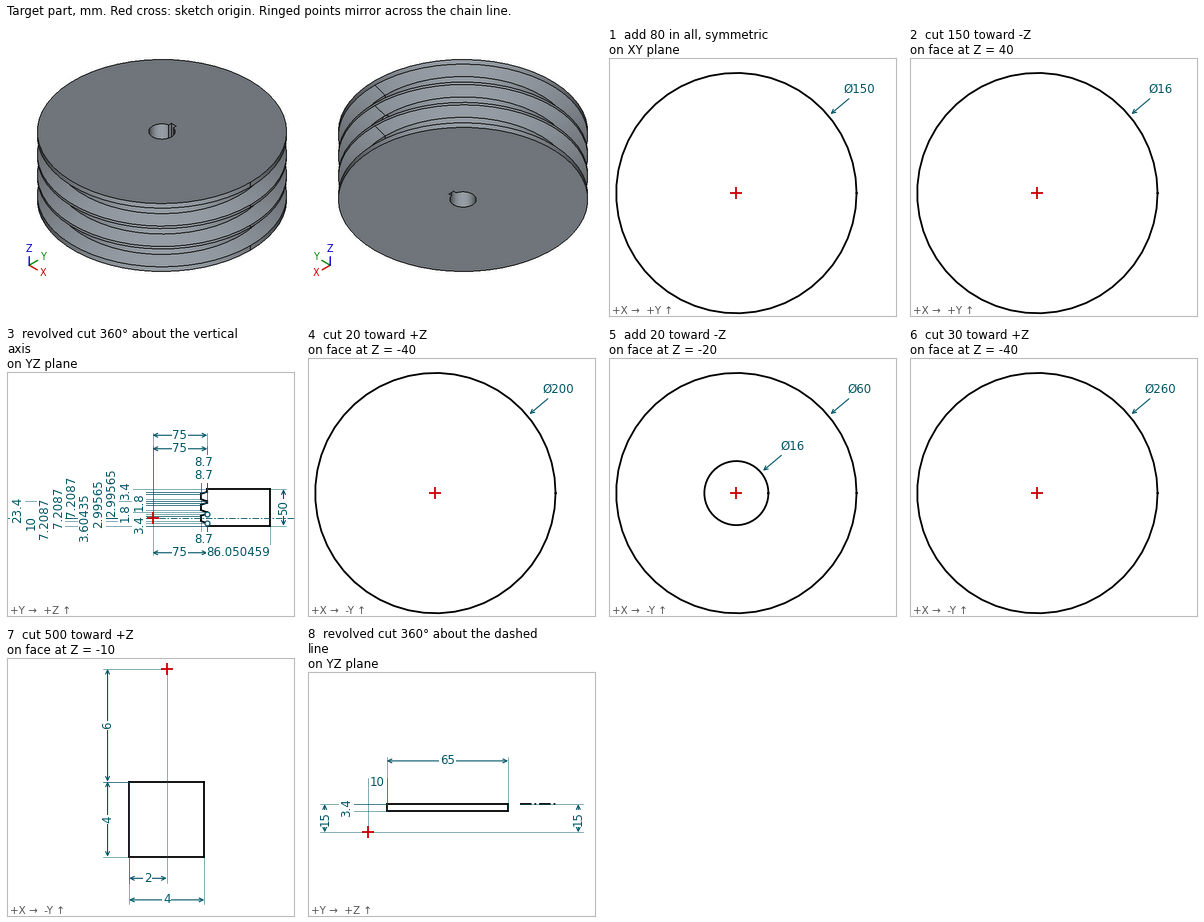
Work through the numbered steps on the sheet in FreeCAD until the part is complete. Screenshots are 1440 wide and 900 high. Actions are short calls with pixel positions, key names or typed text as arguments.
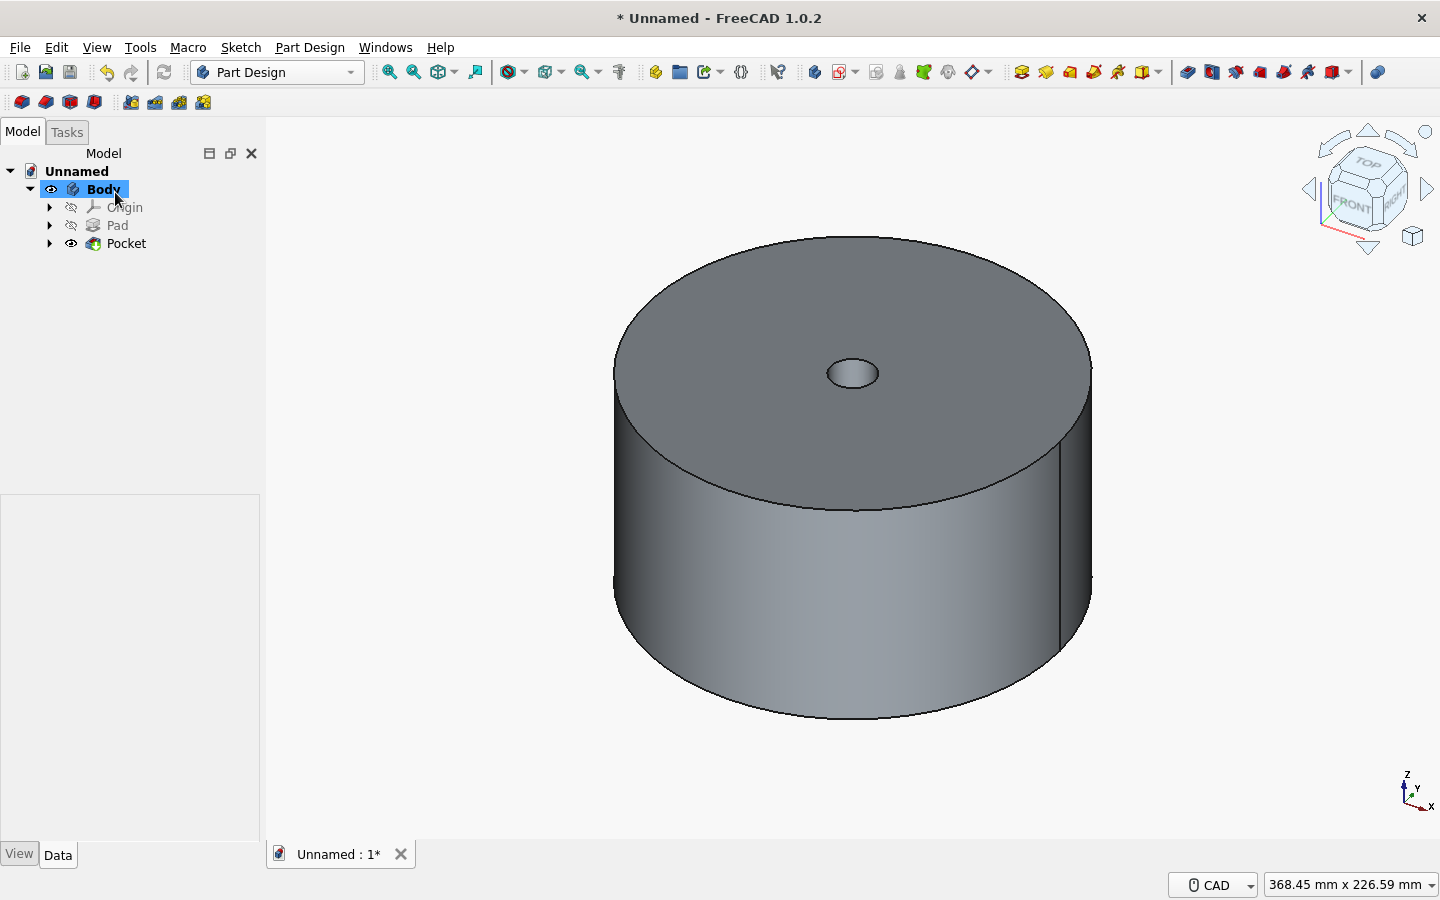
click(840, 72)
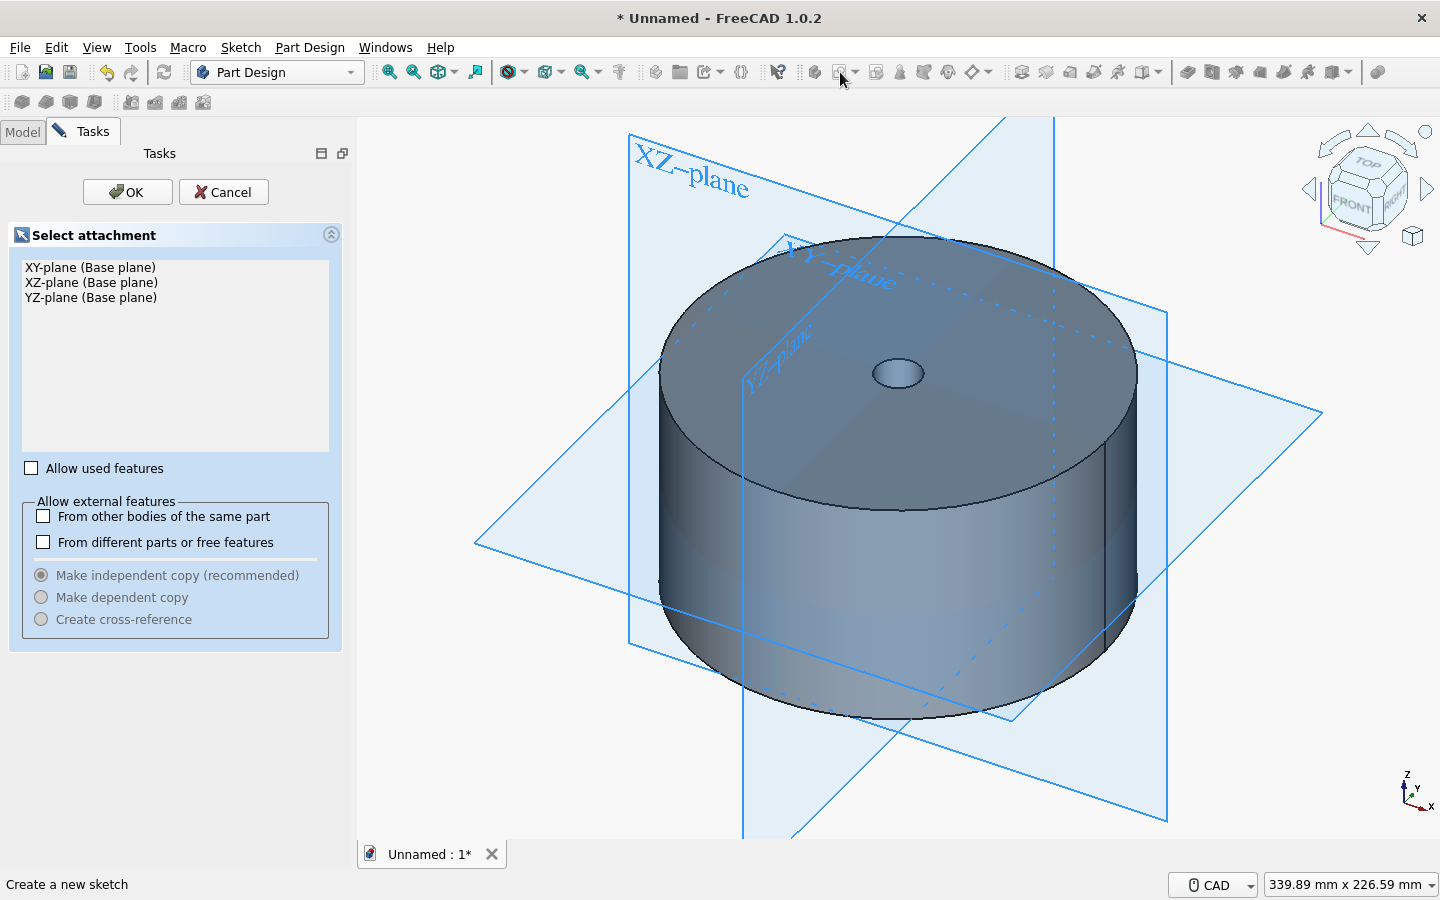
click(82, 298)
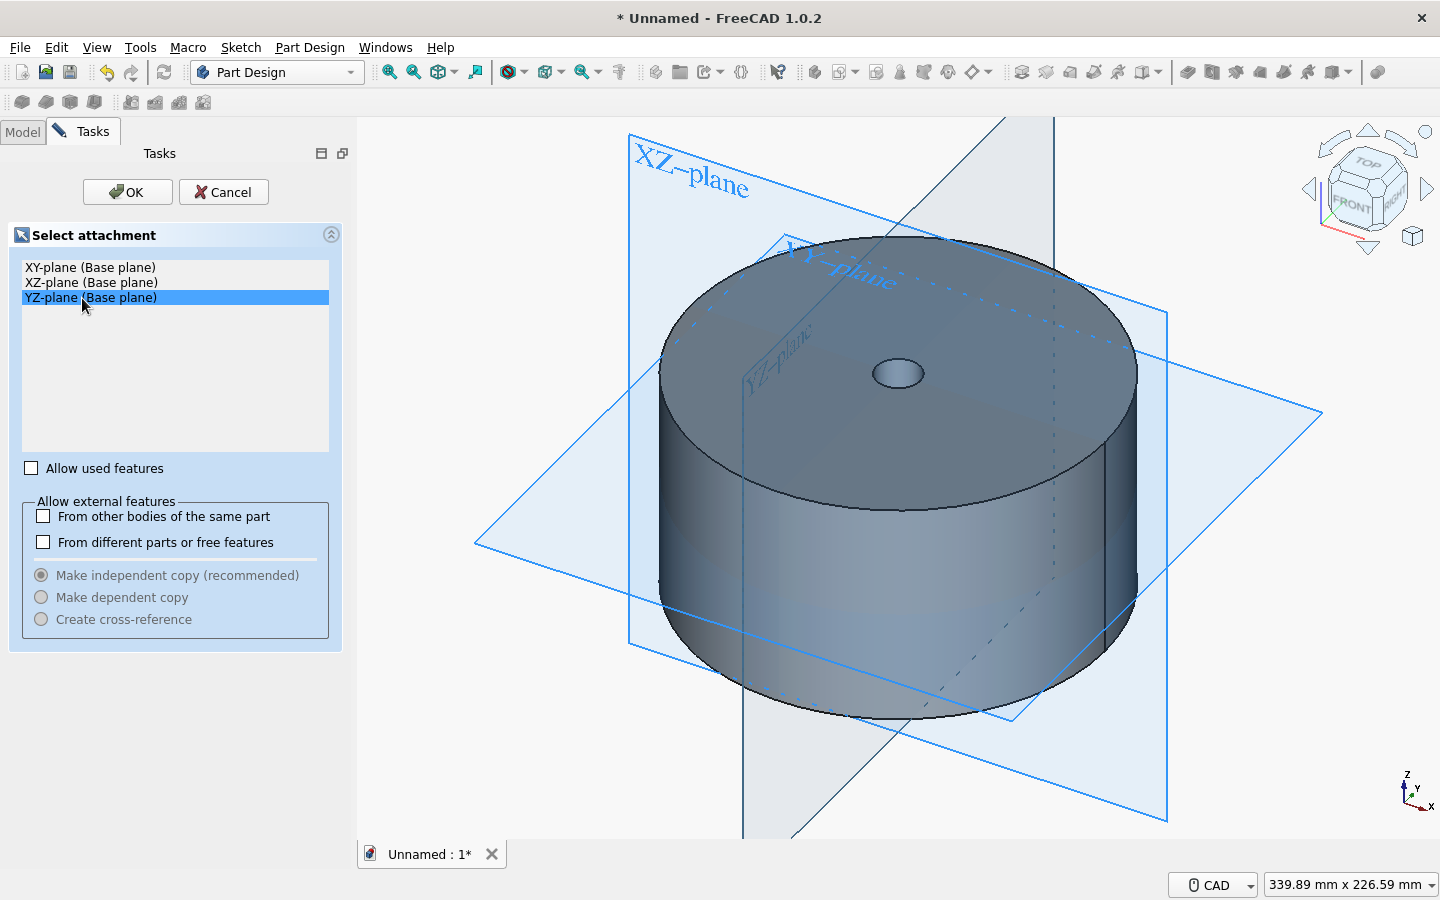
click(128, 192)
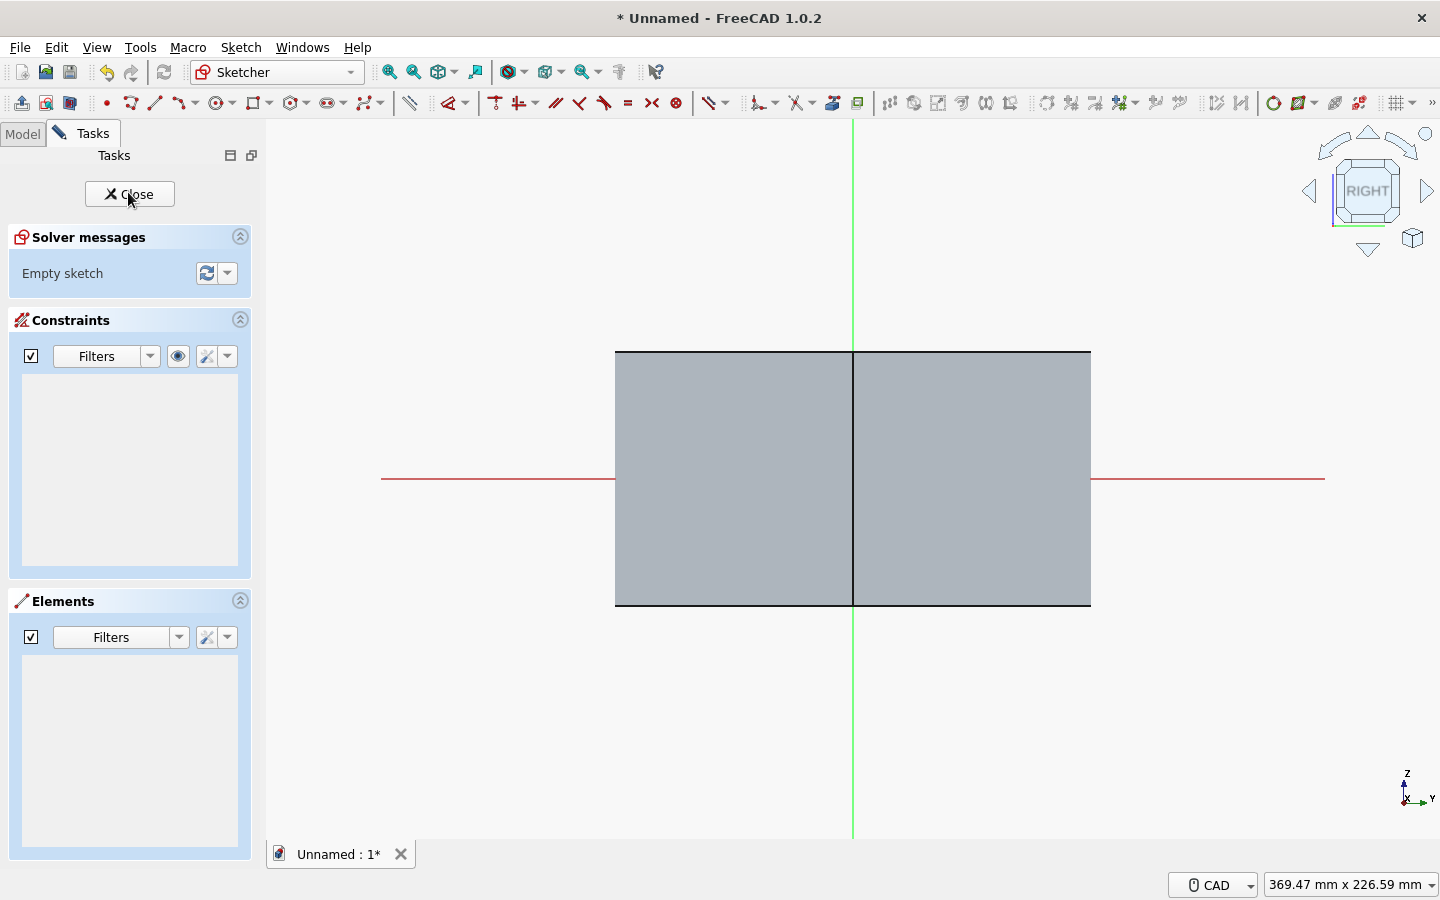
click(70, 104)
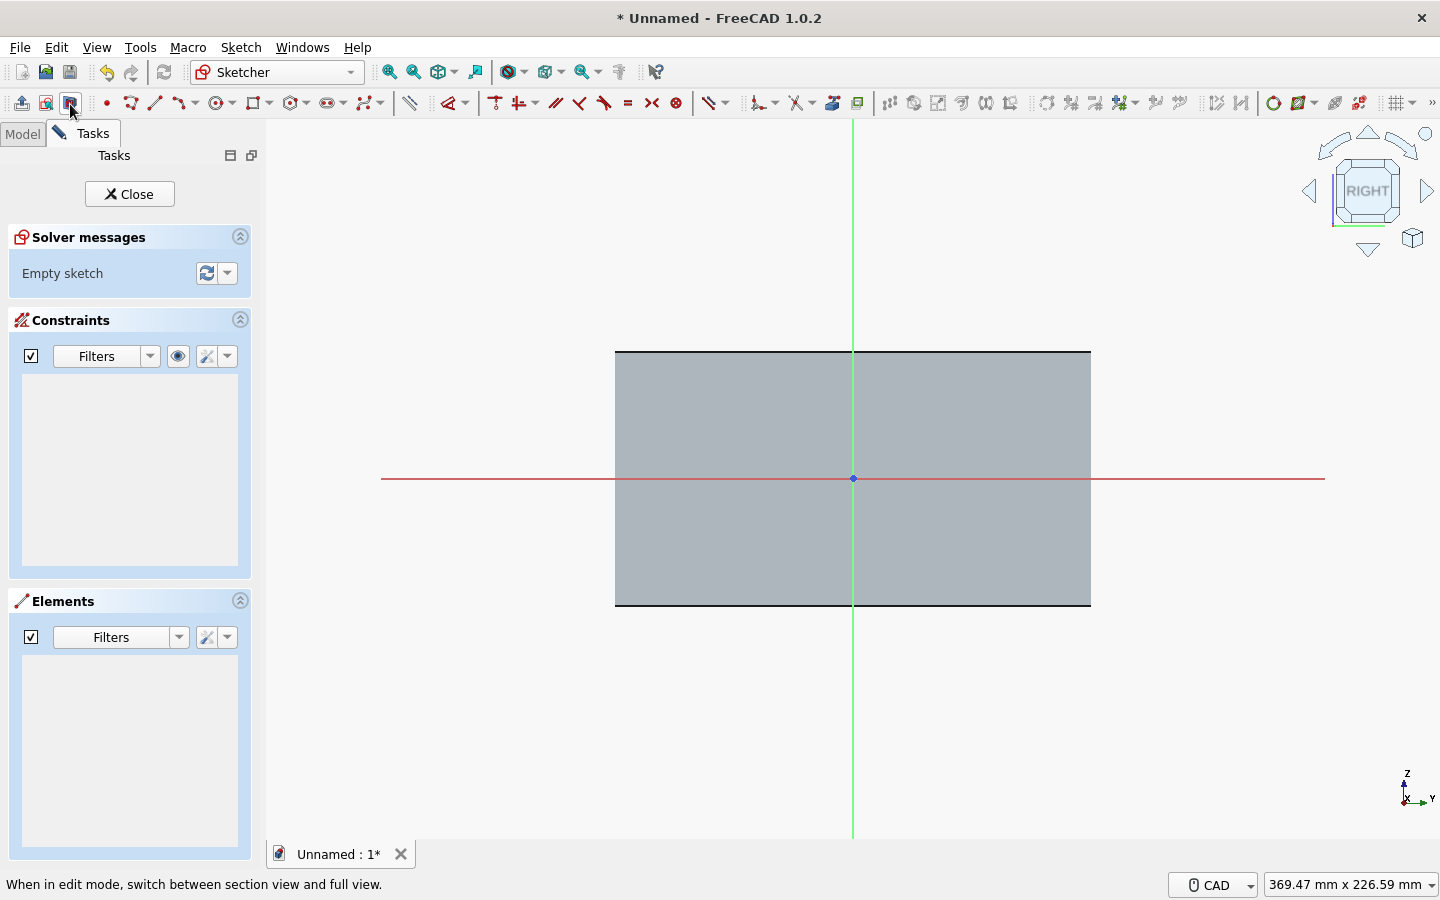
scroll(294, 694, down, 1)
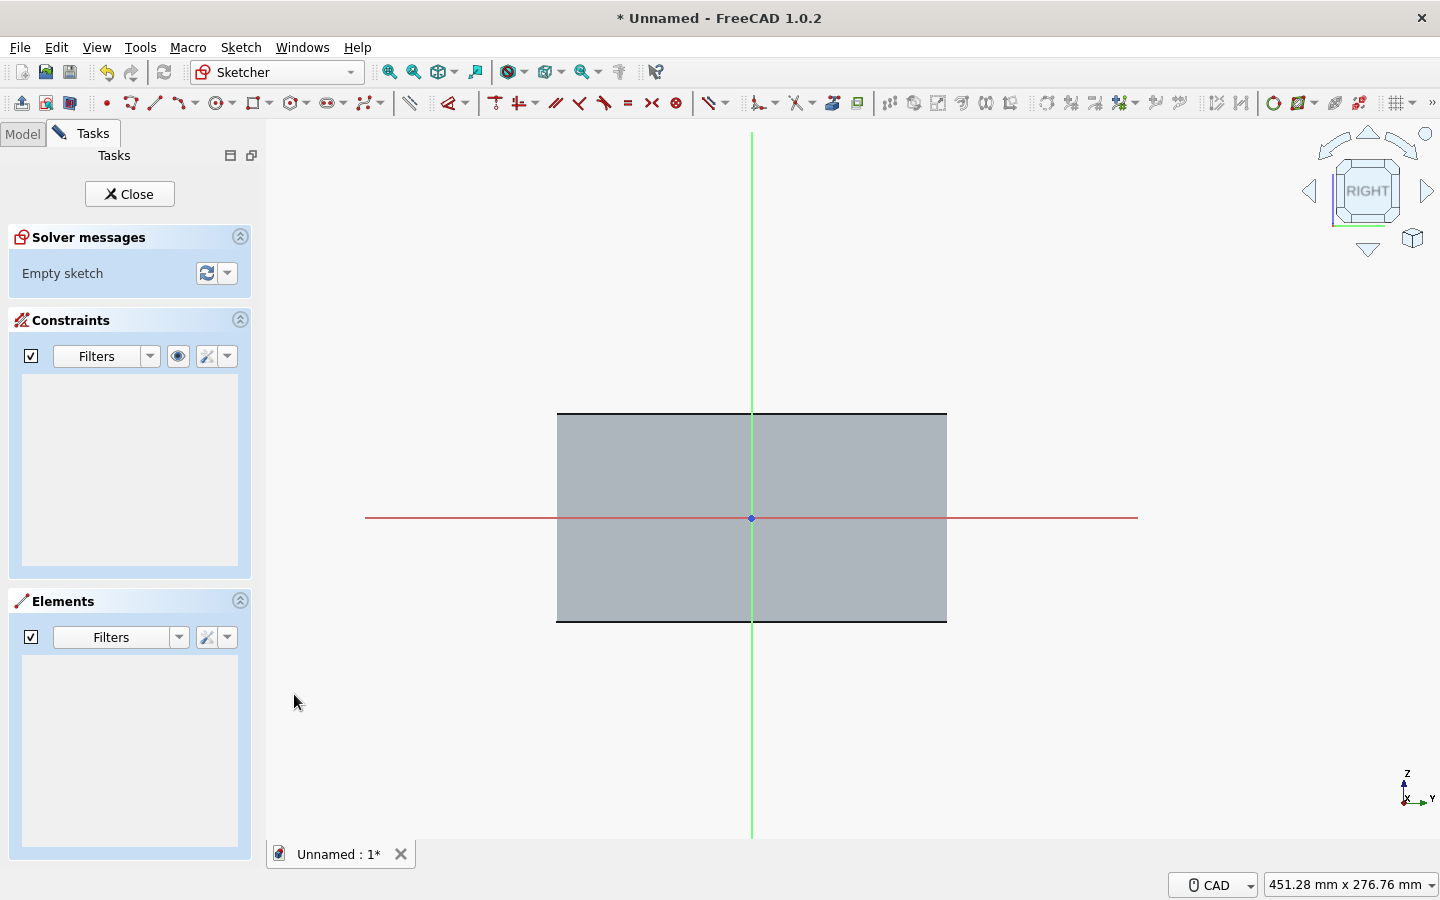
scroll(1176, 479, up, 3)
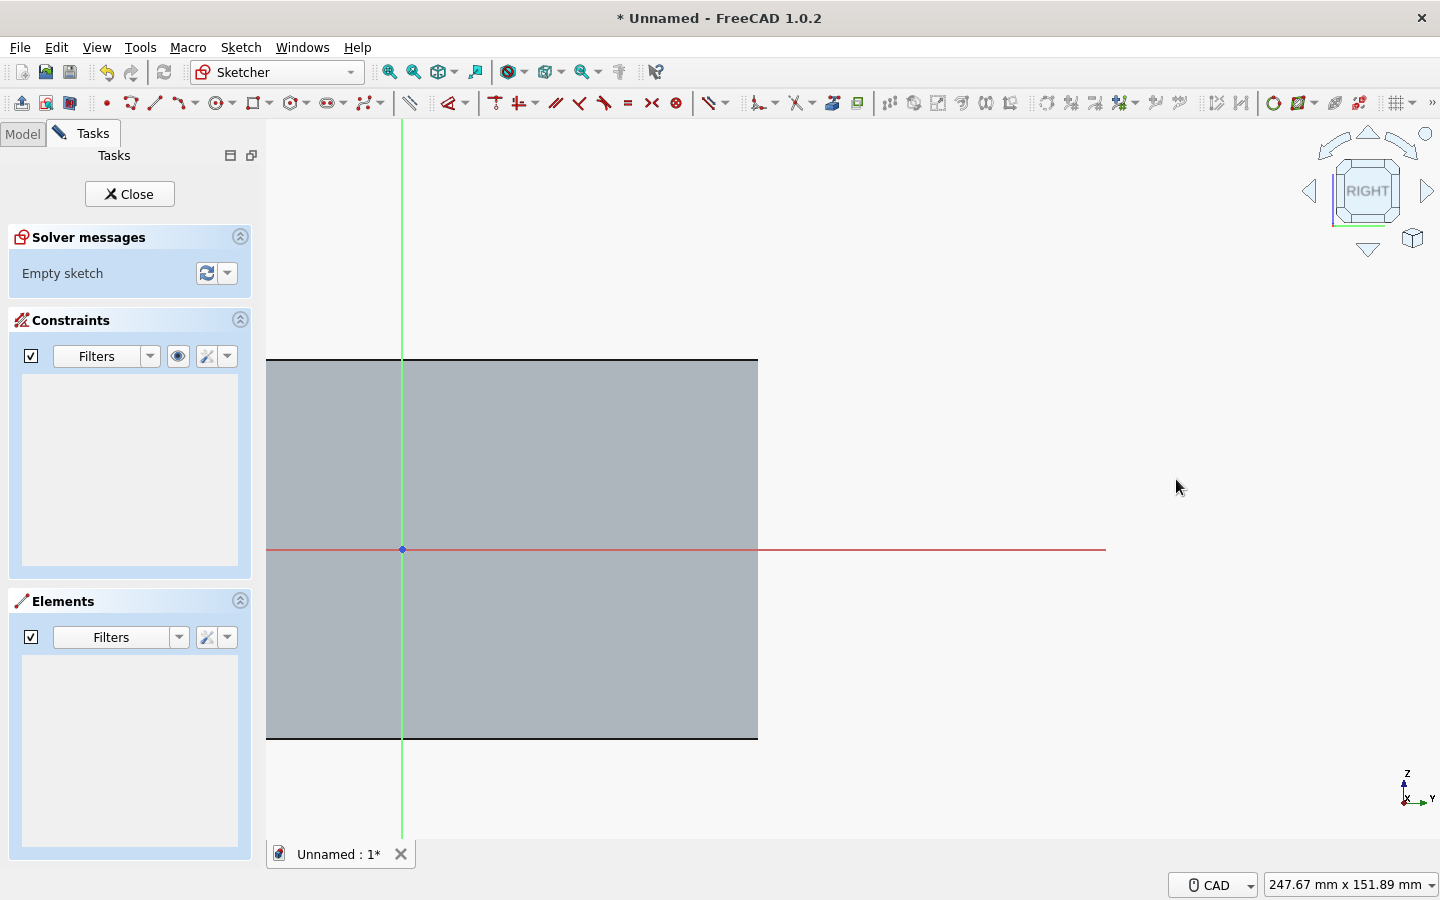
key(g)
key(m)